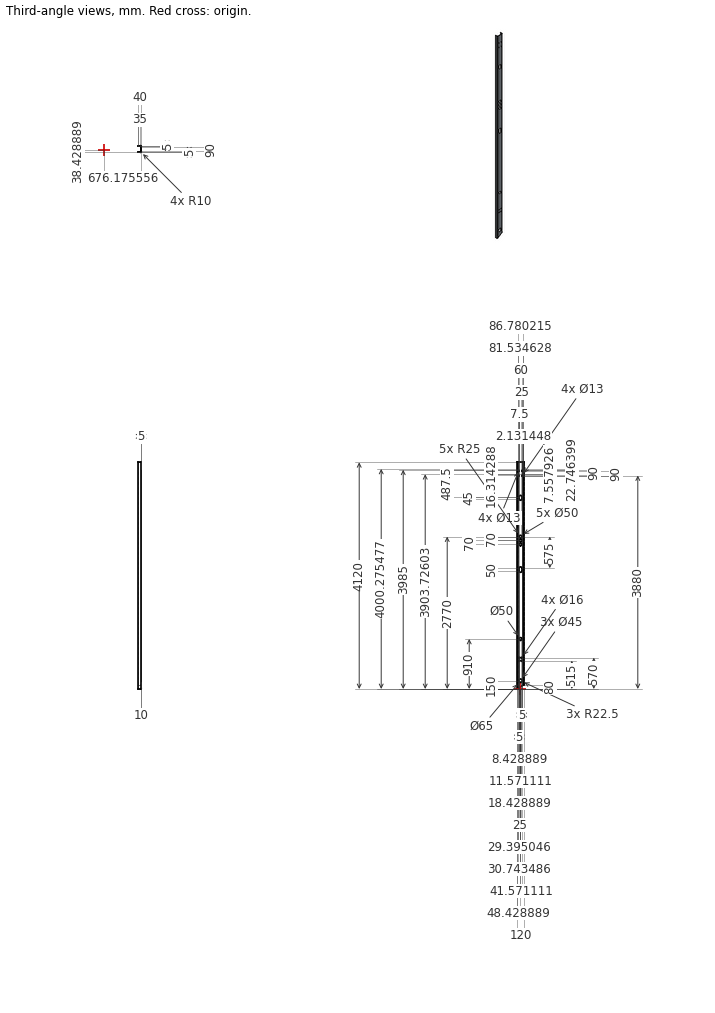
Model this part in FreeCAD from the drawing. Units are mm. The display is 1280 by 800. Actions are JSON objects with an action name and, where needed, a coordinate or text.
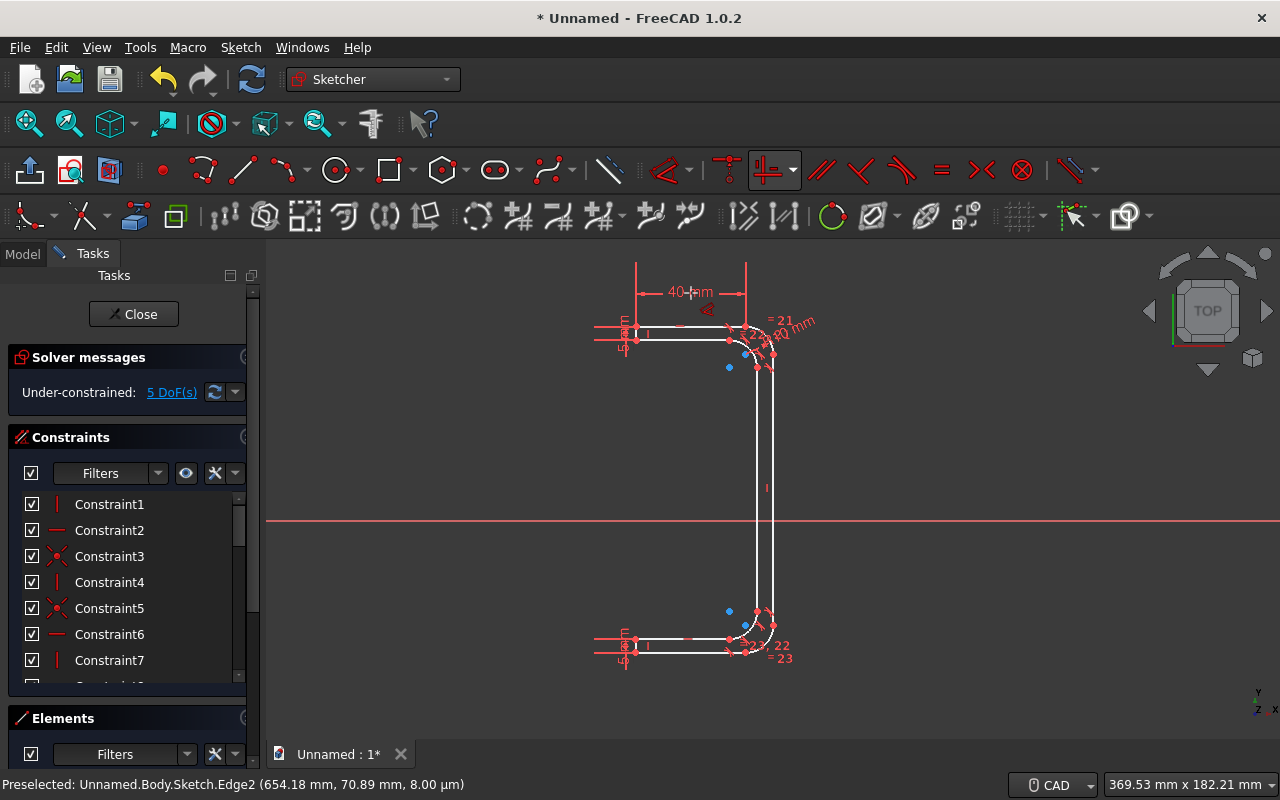
{"action": "left_click", "coordinate": [664, 340]}
{"action": "left_click", "coordinate": [683, 374]}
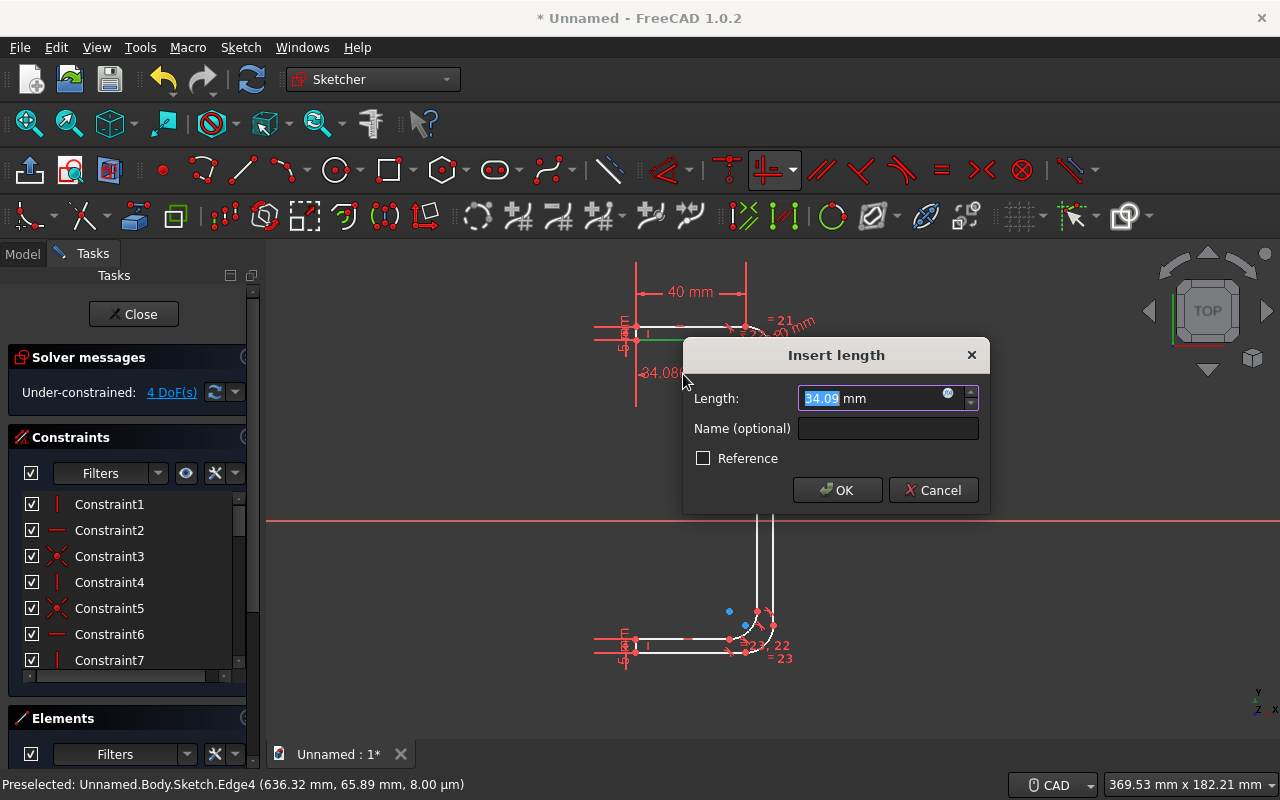
{"action": "type", "text": "35"}
{"action": "key", "text": "Return"}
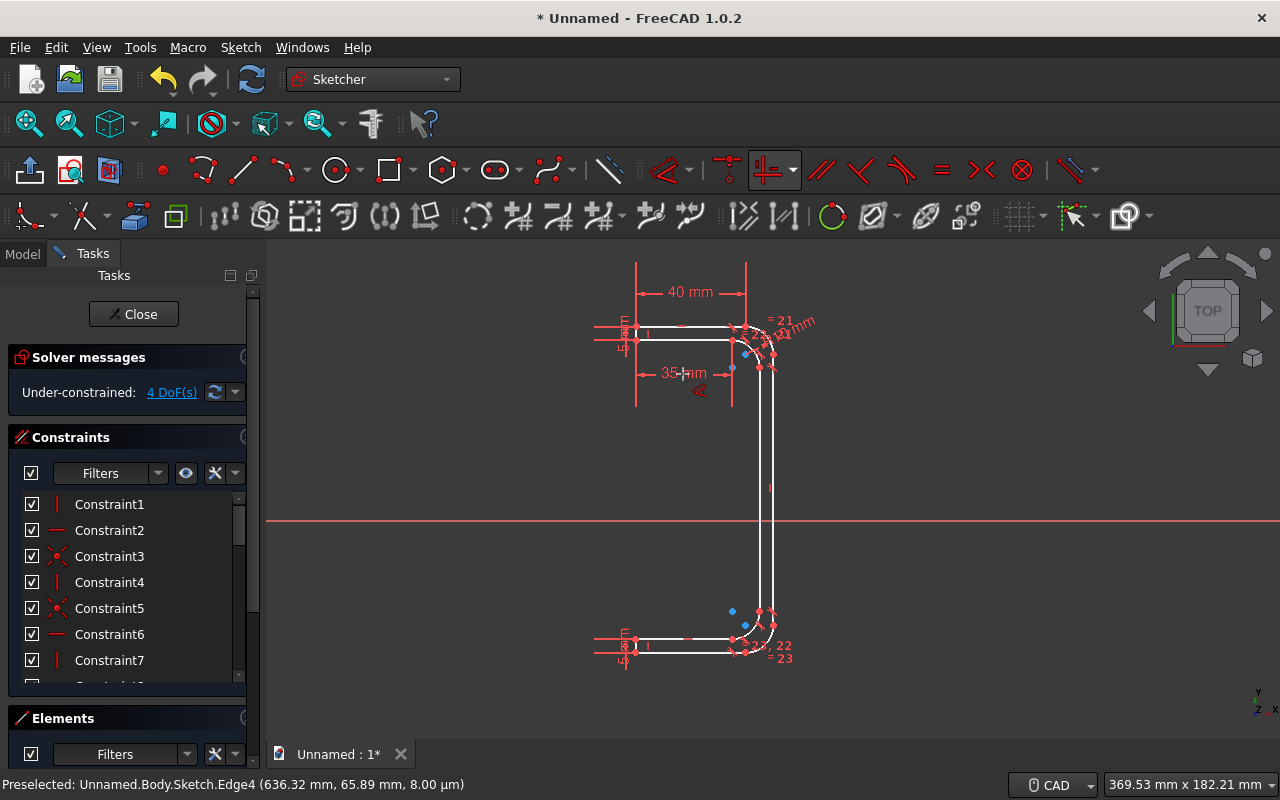
{"action": "left_click", "coordinate": [760, 441]}
{"action": "left_click", "coordinate": [794, 490]}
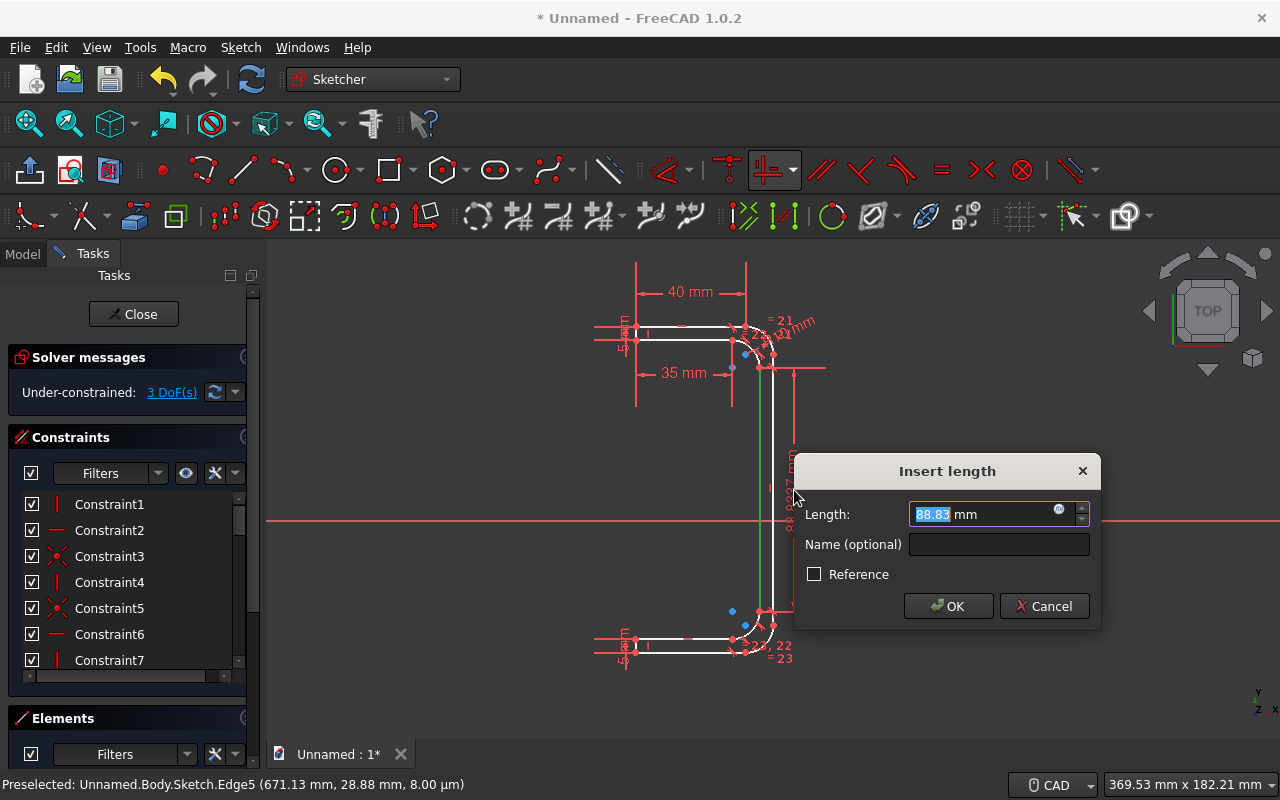
{"action": "type", "text": "90"}
{"action": "key", "text": "Return"}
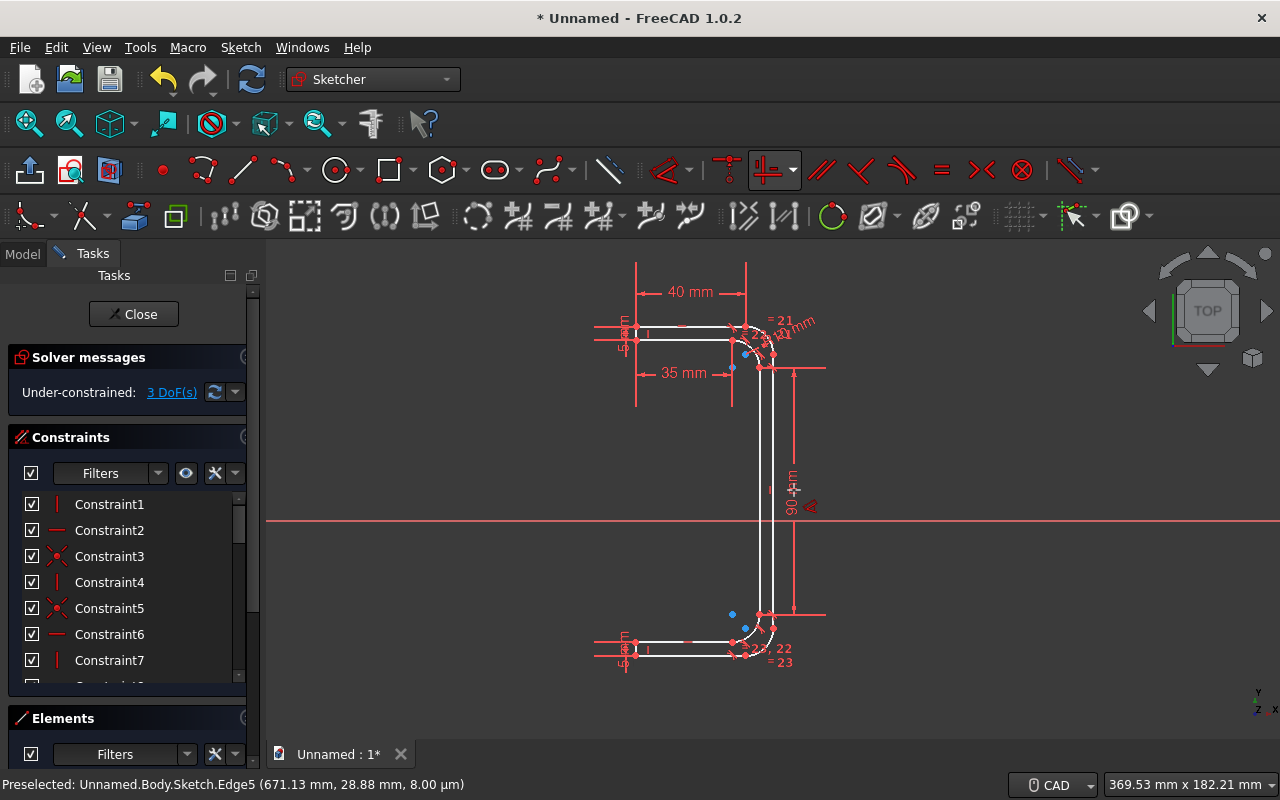
{"action": "left_click", "coordinate": [703, 642]}
{"action": "left_click", "coordinate": [684, 676]}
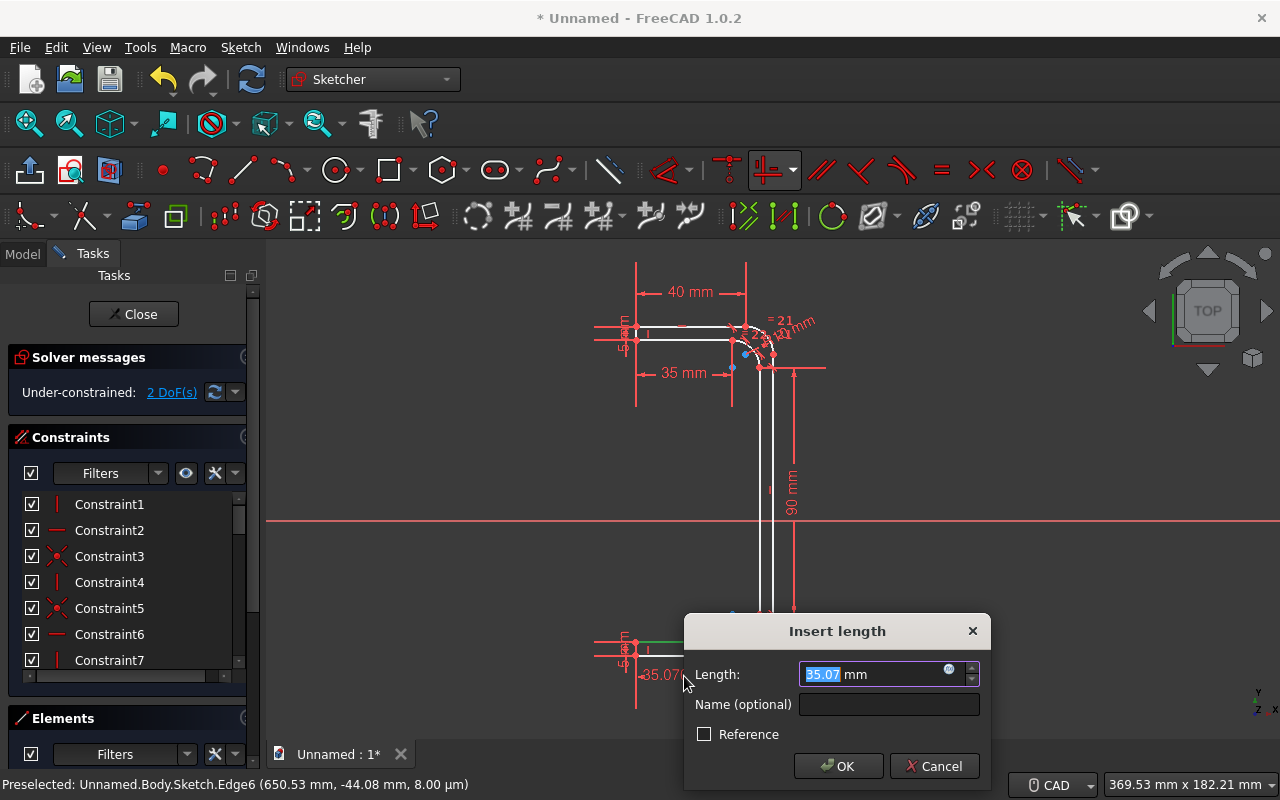
{"action": "type", "text": "35"}
{"action": "key", "text": "Return"}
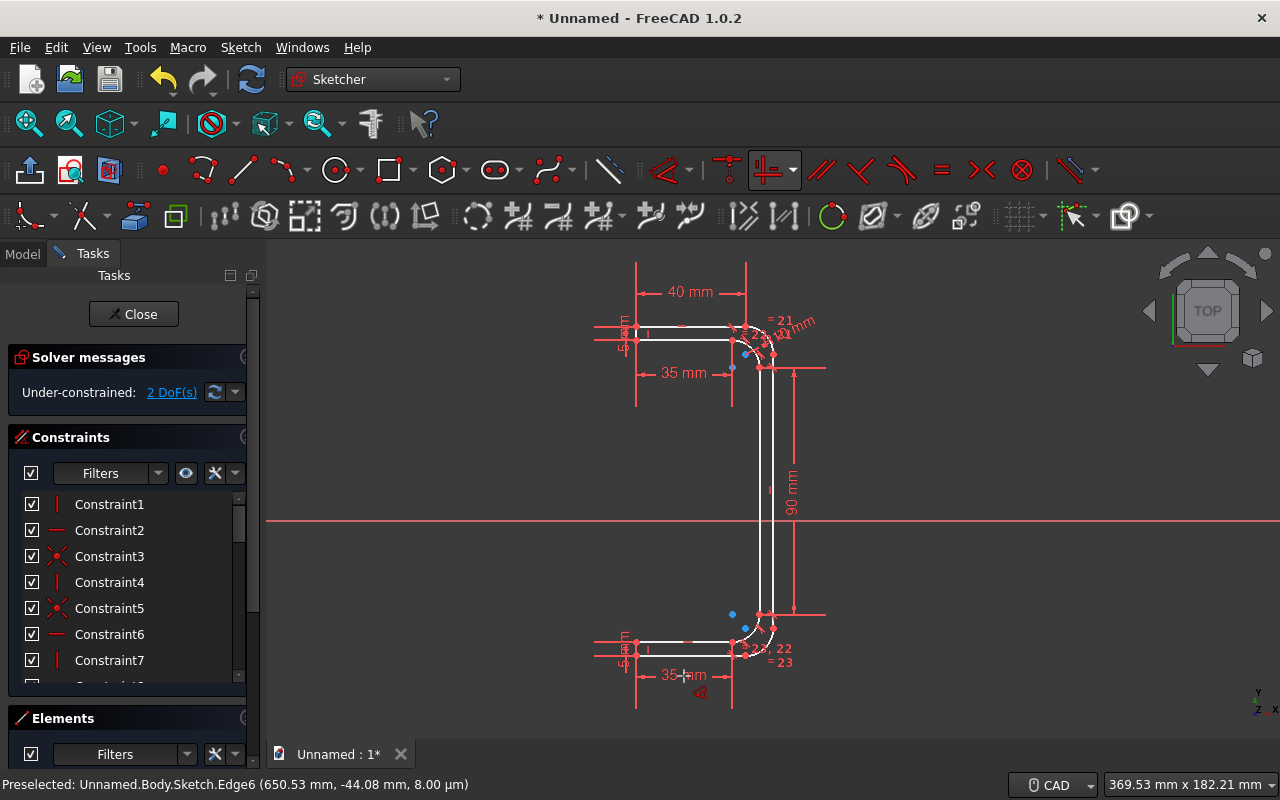
{"action": "left_click", "coordinate": [773, 628]}
{"action": "left_click", "coordinate": [807, 575]}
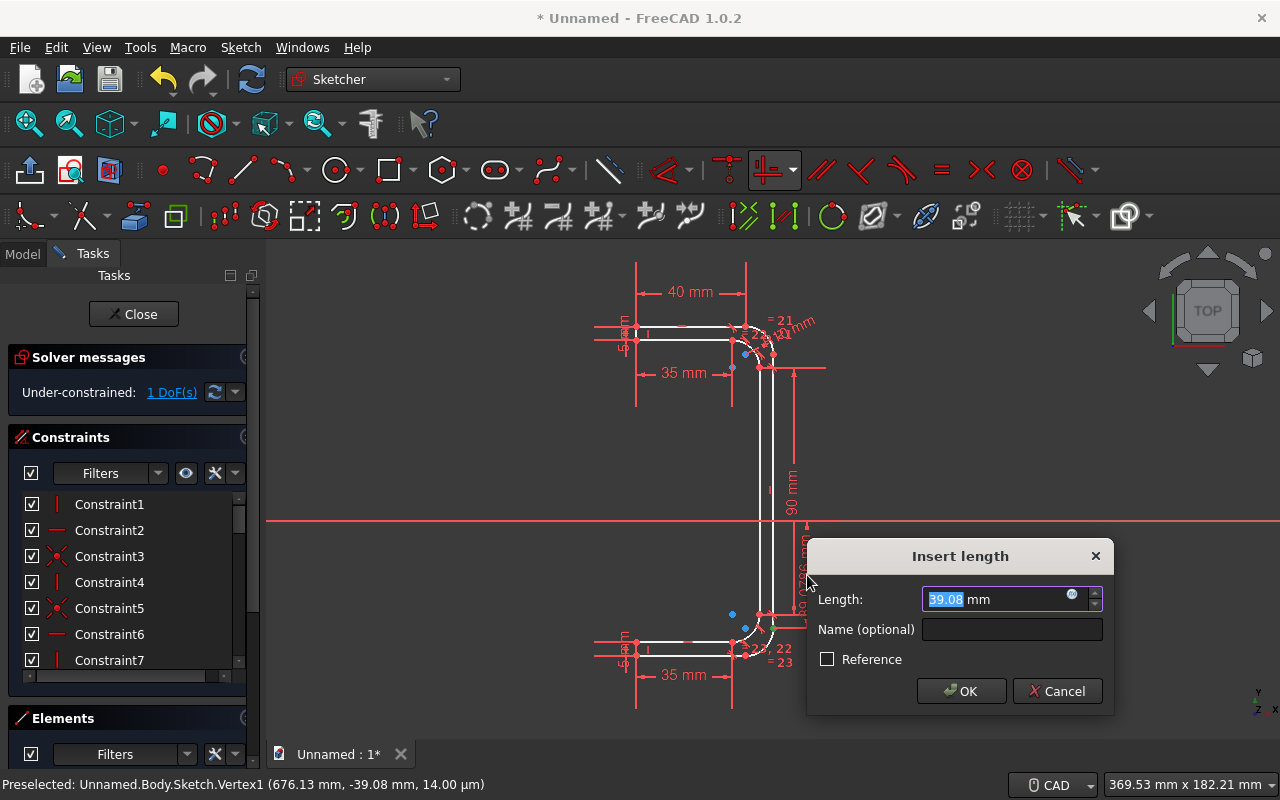
{"action": "type", "text": "38.428889"}
{"action": "key", "text": "Return"}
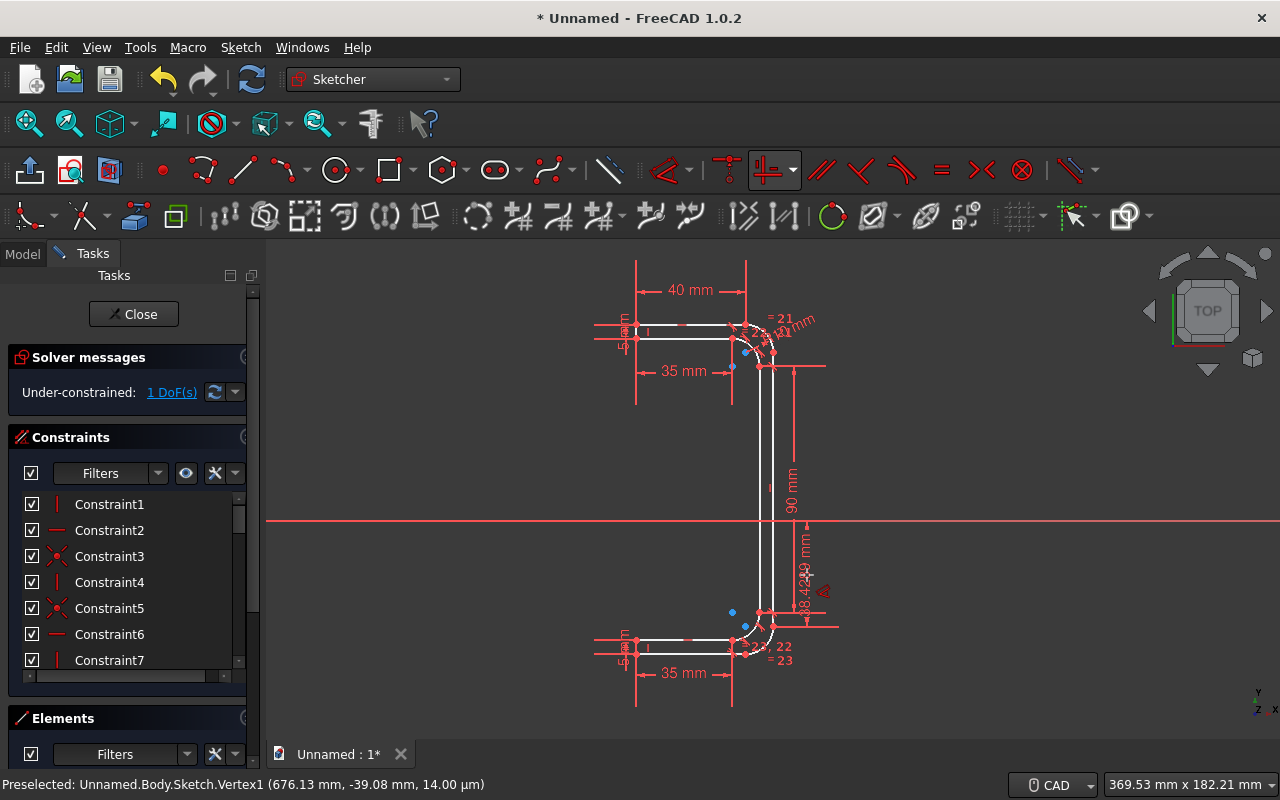
{"action": "left_click", "coordinate": [773, 627]}
{"action": "left_click", "coordinate": [534, 661]}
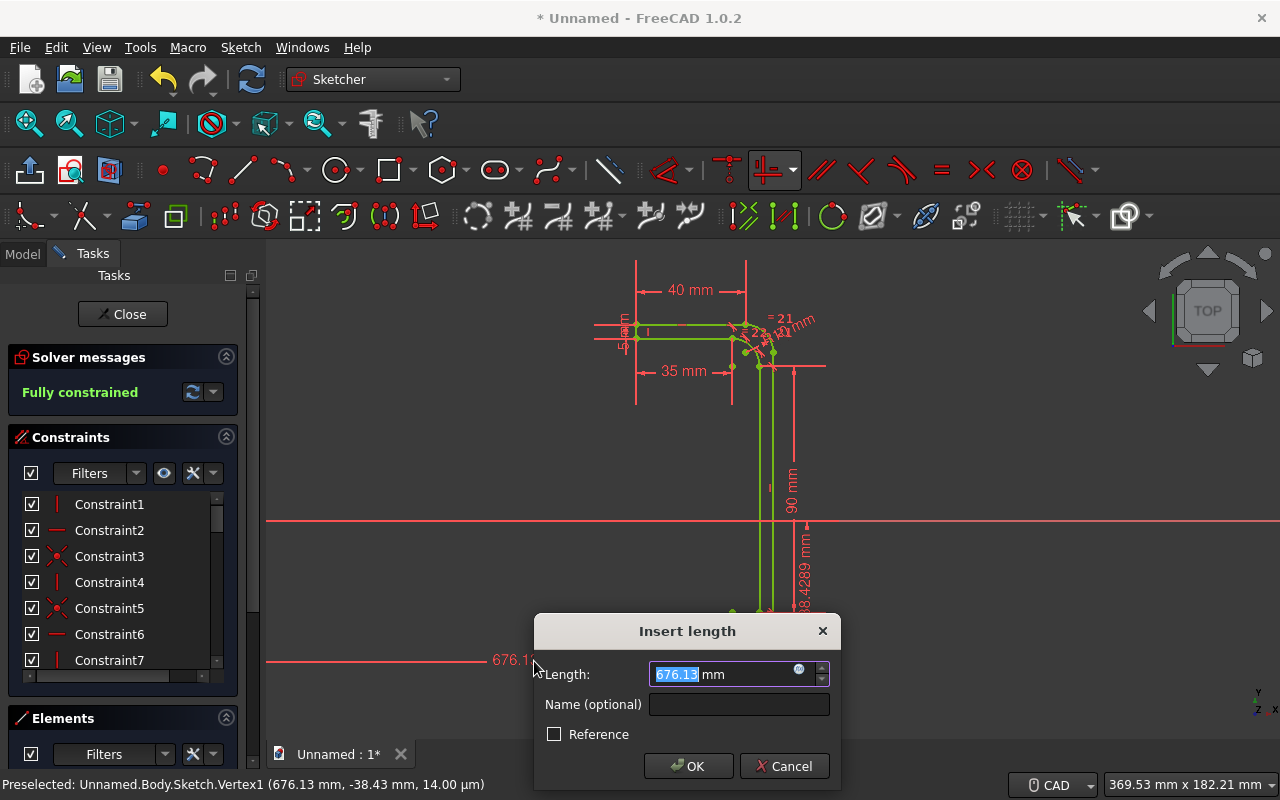
{"action": "type", "text": "676.175556"}
{"action": "key", "text": "Return"}
{"action": "key", "text": "Escape"}